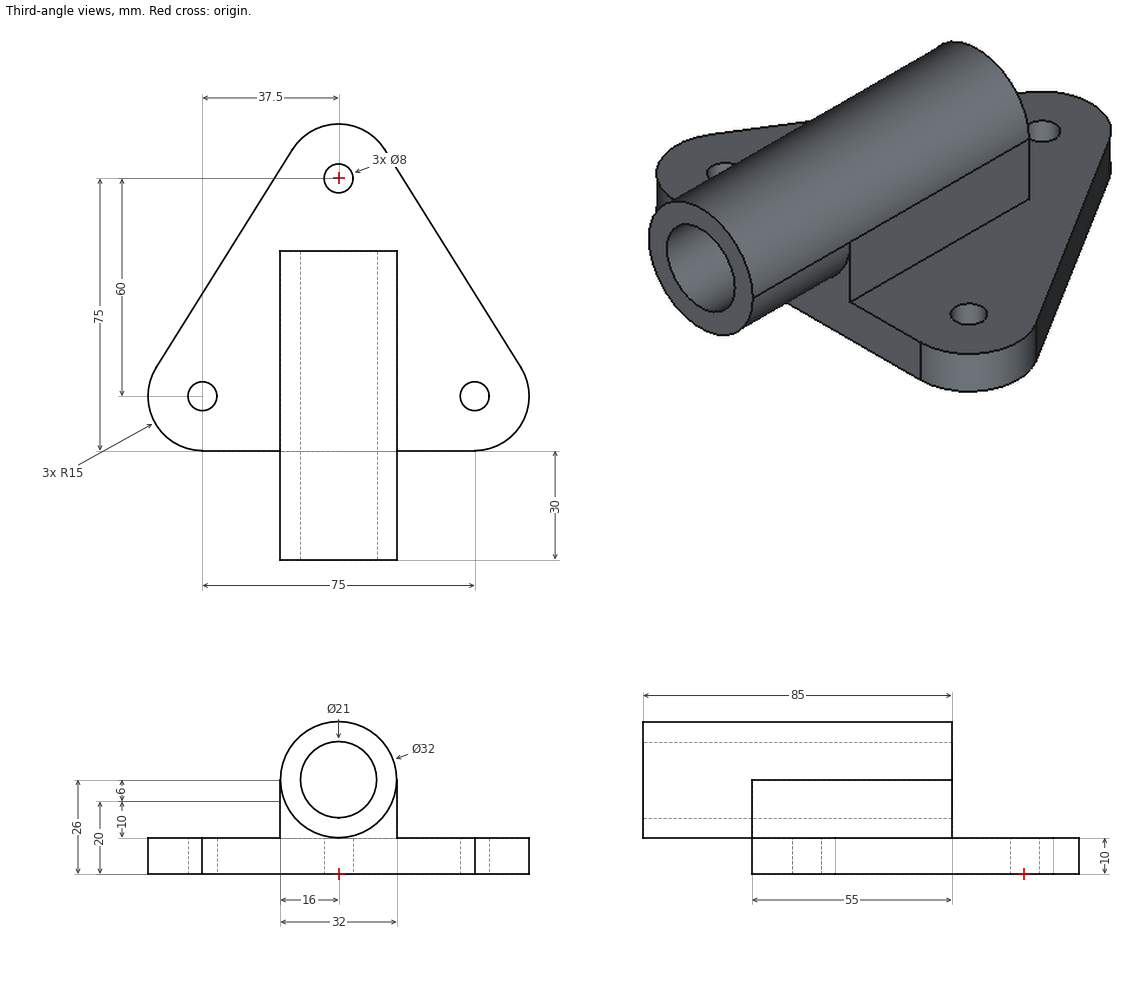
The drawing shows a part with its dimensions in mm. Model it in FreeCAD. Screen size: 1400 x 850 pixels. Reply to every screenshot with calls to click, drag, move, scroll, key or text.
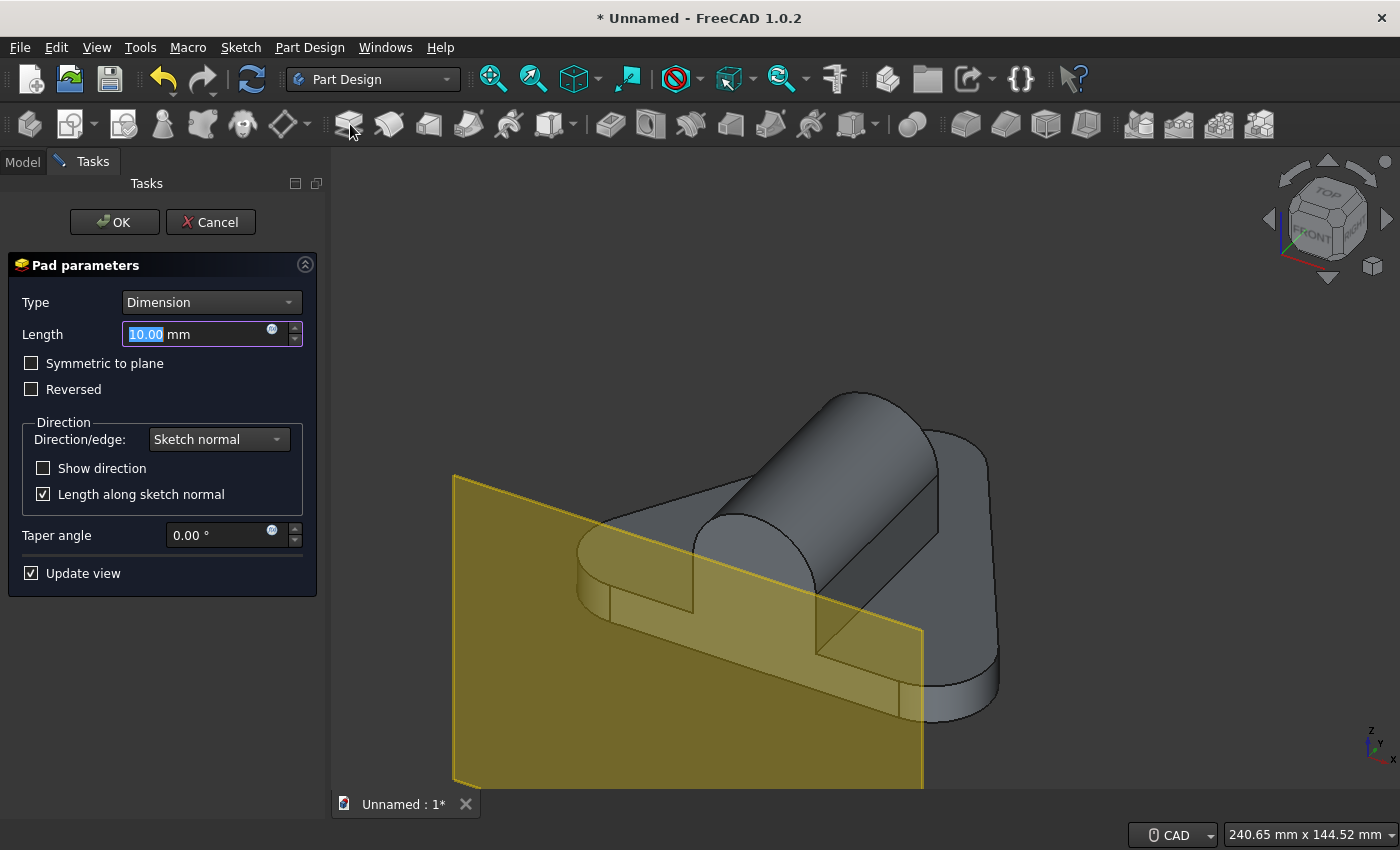
text(30)
key(Tab)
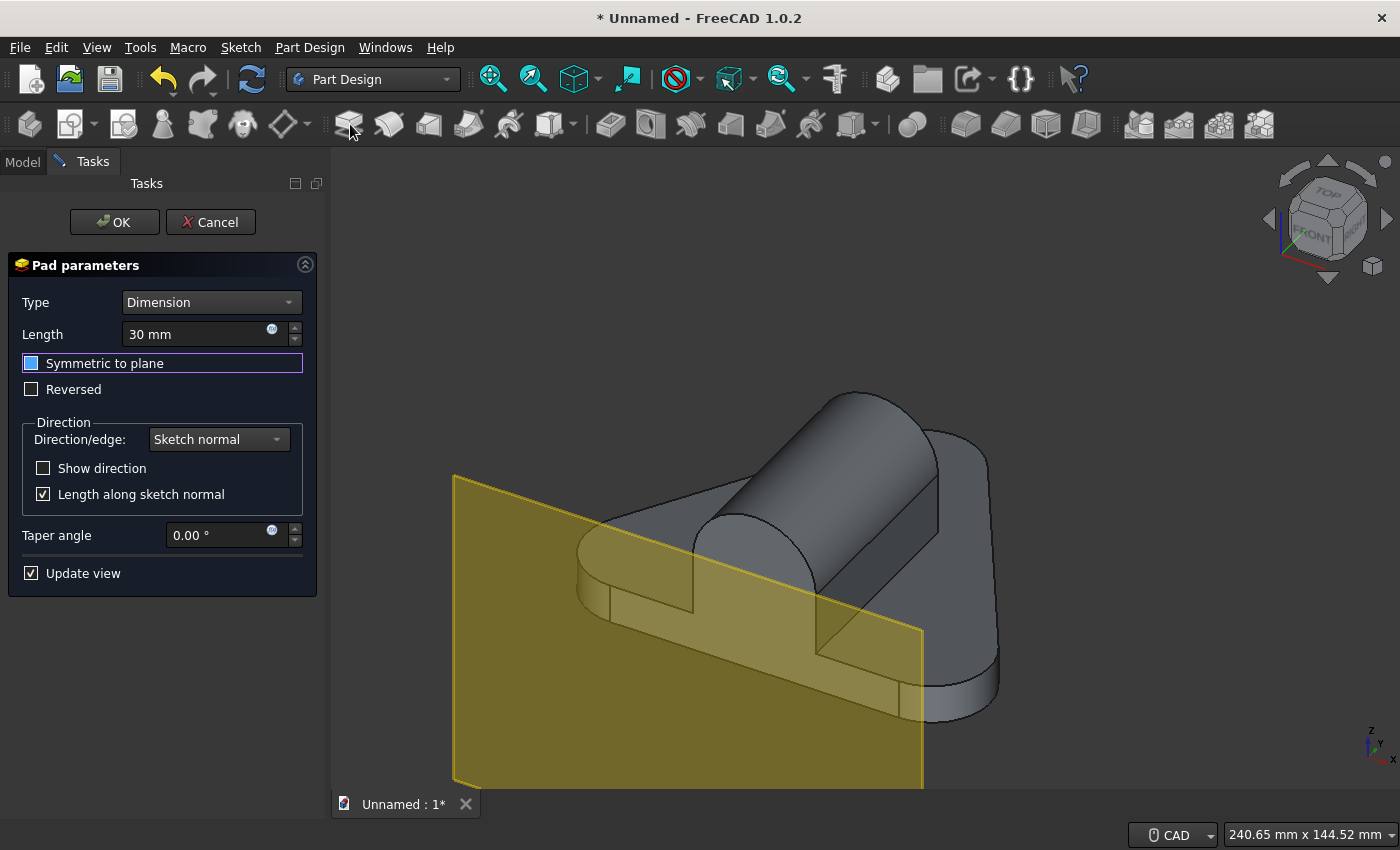
click(30, 389)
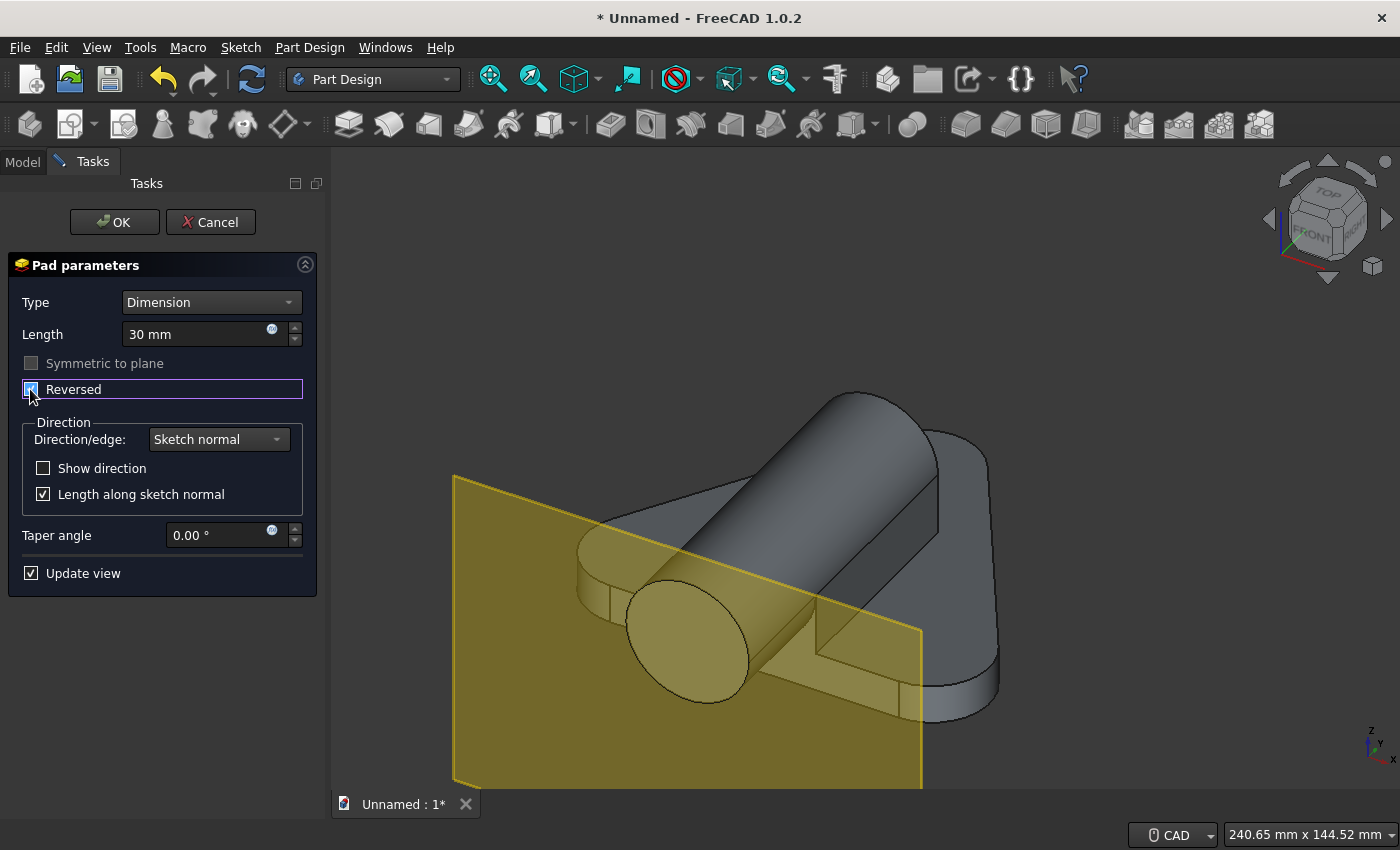
click(115, 222)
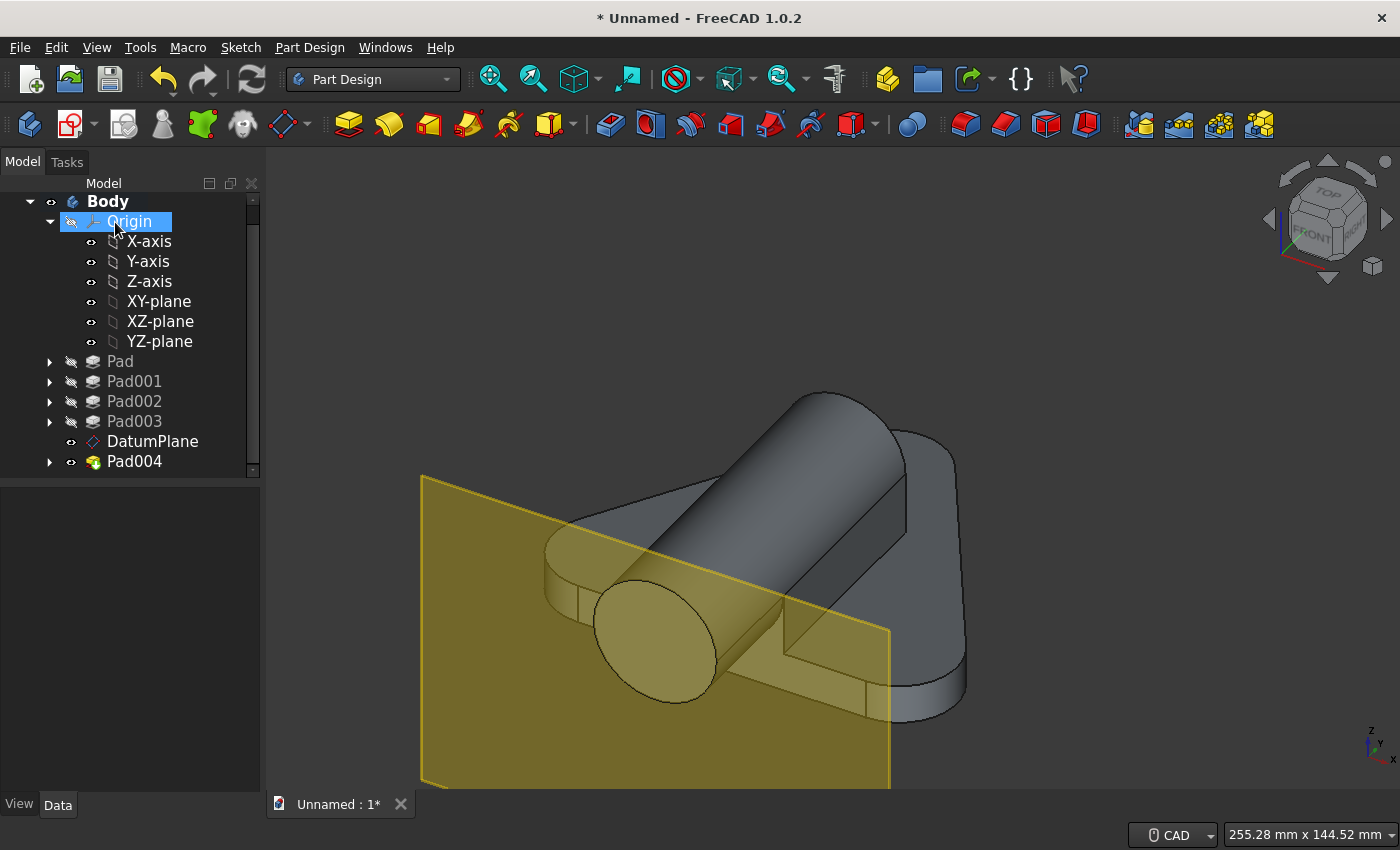
click(116, 442)
key(space)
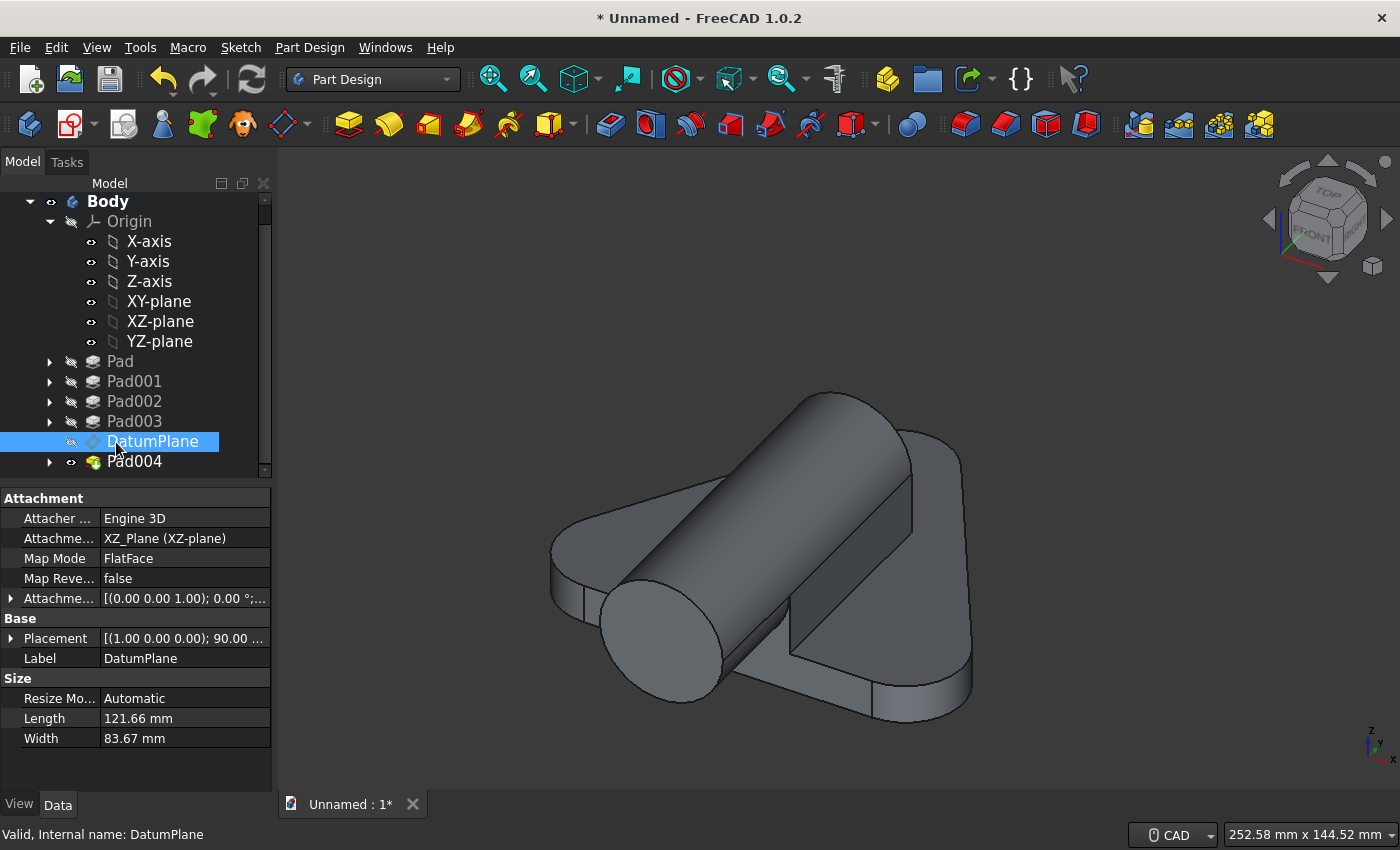
click(494, 80)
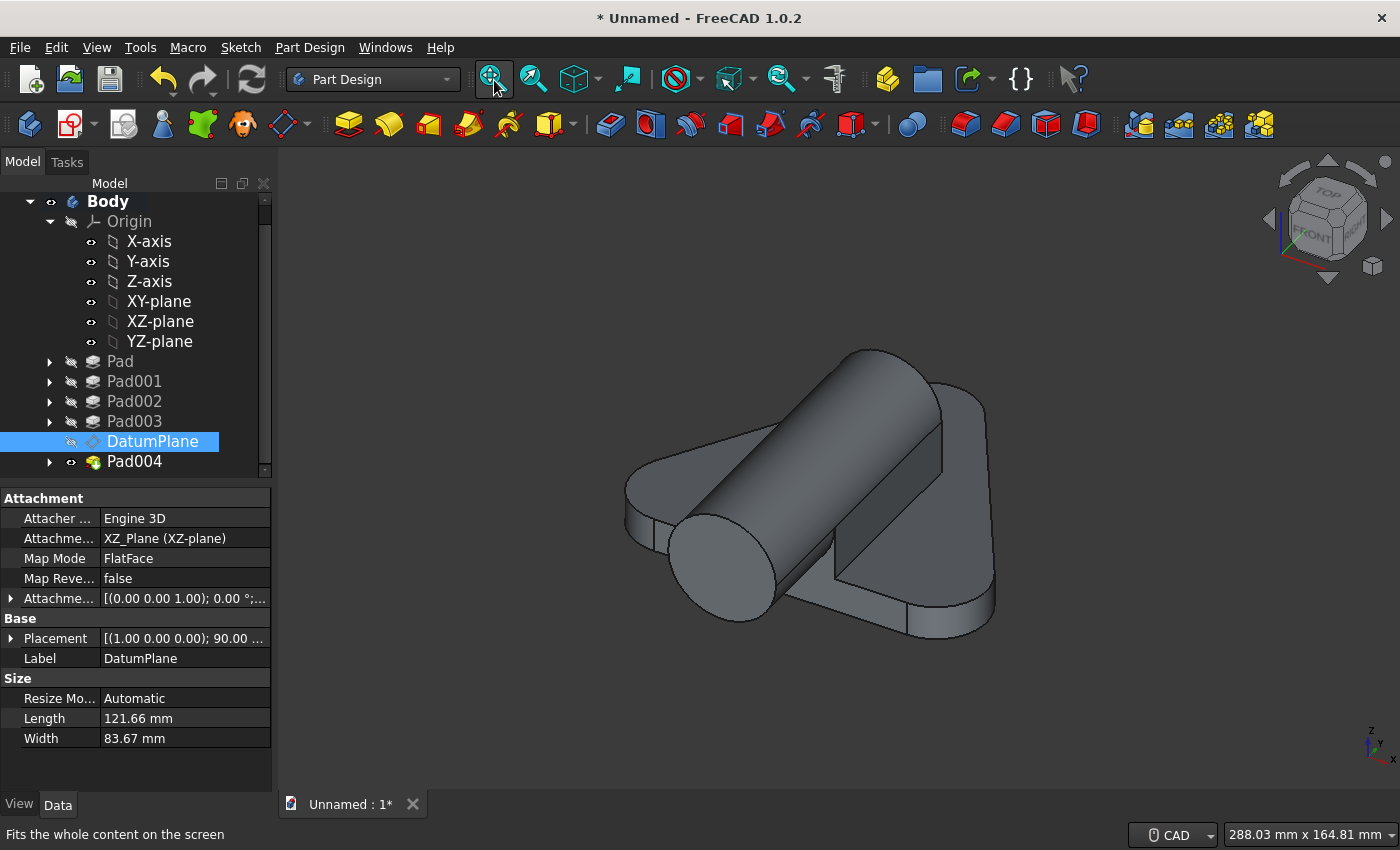
click(722, 567)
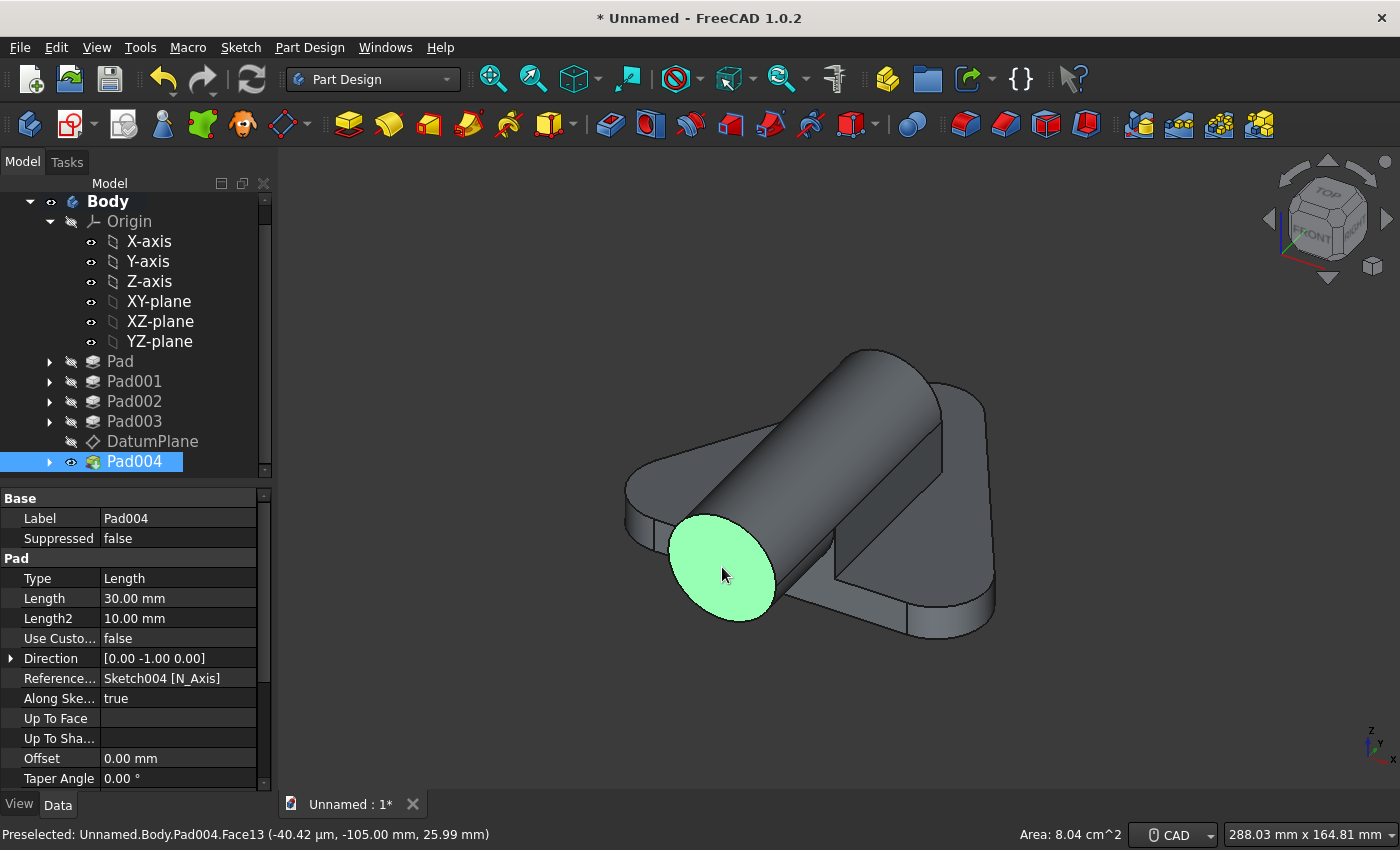
click(70, 124)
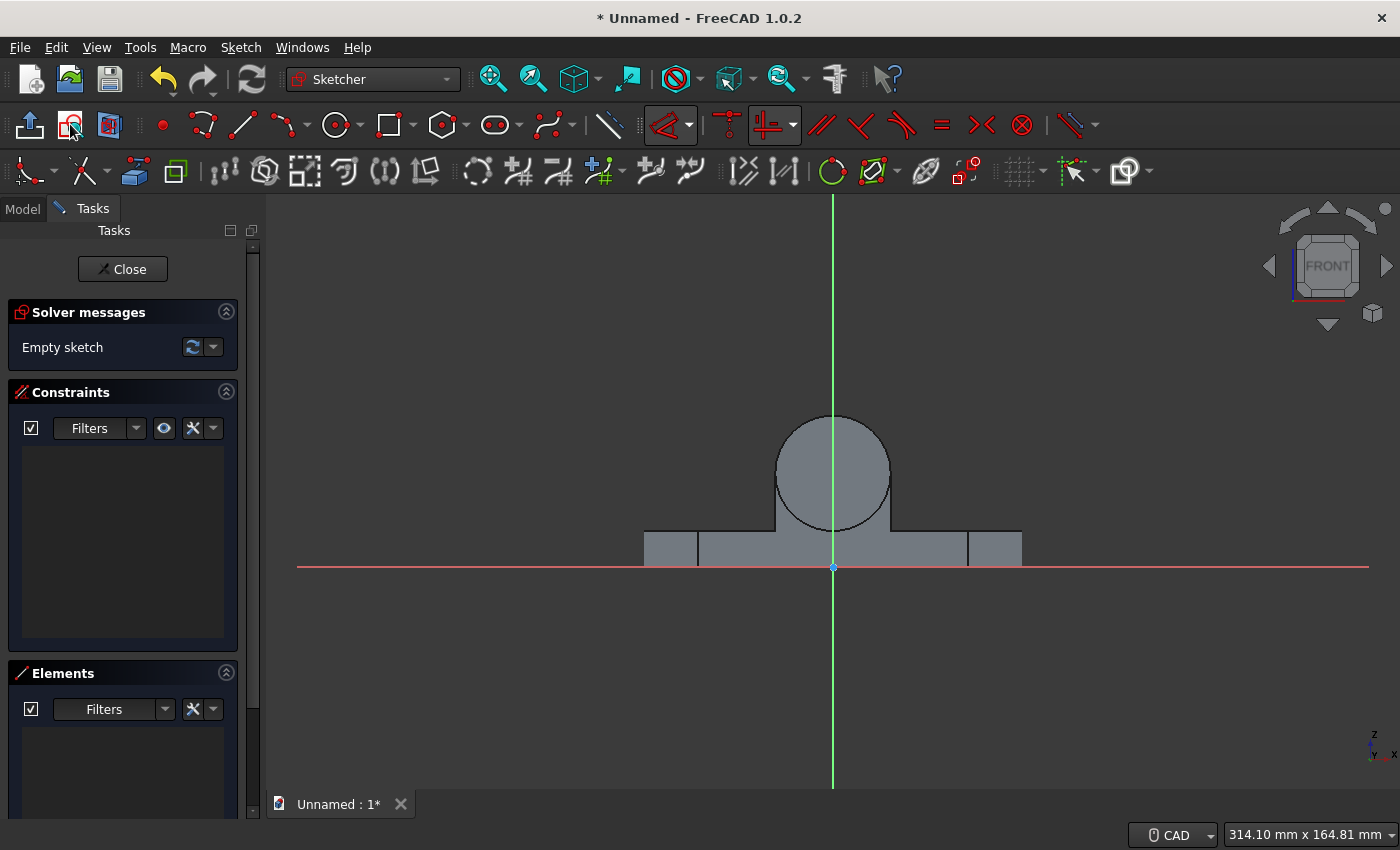
scroll(873, 507, up, 5)